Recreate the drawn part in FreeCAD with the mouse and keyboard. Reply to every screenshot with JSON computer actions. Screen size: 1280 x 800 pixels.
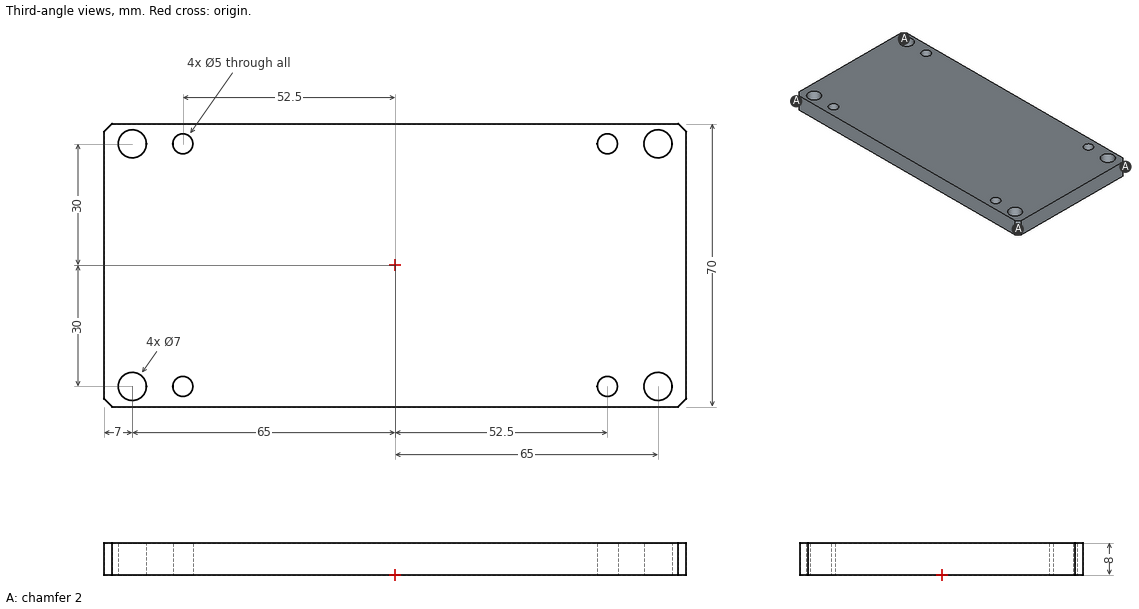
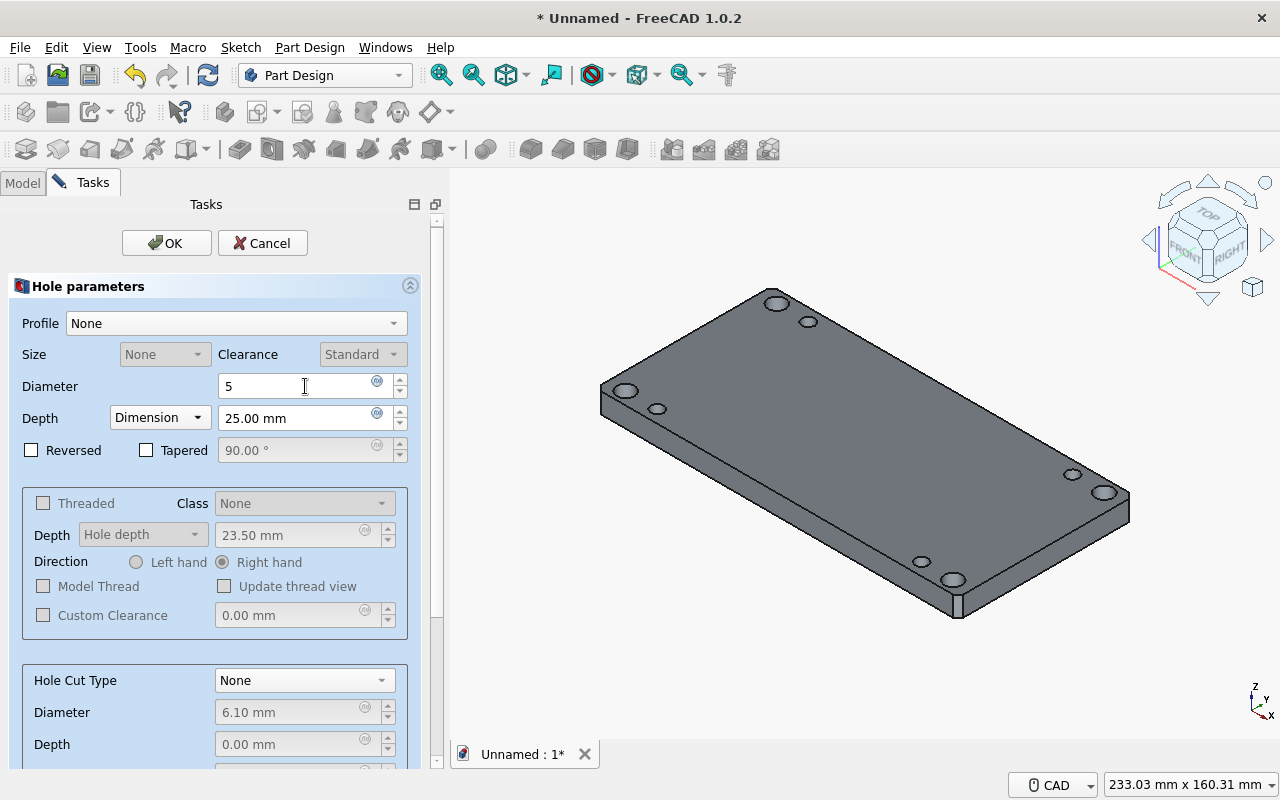
{"action": "left_click", "coordinate": [161, 418]}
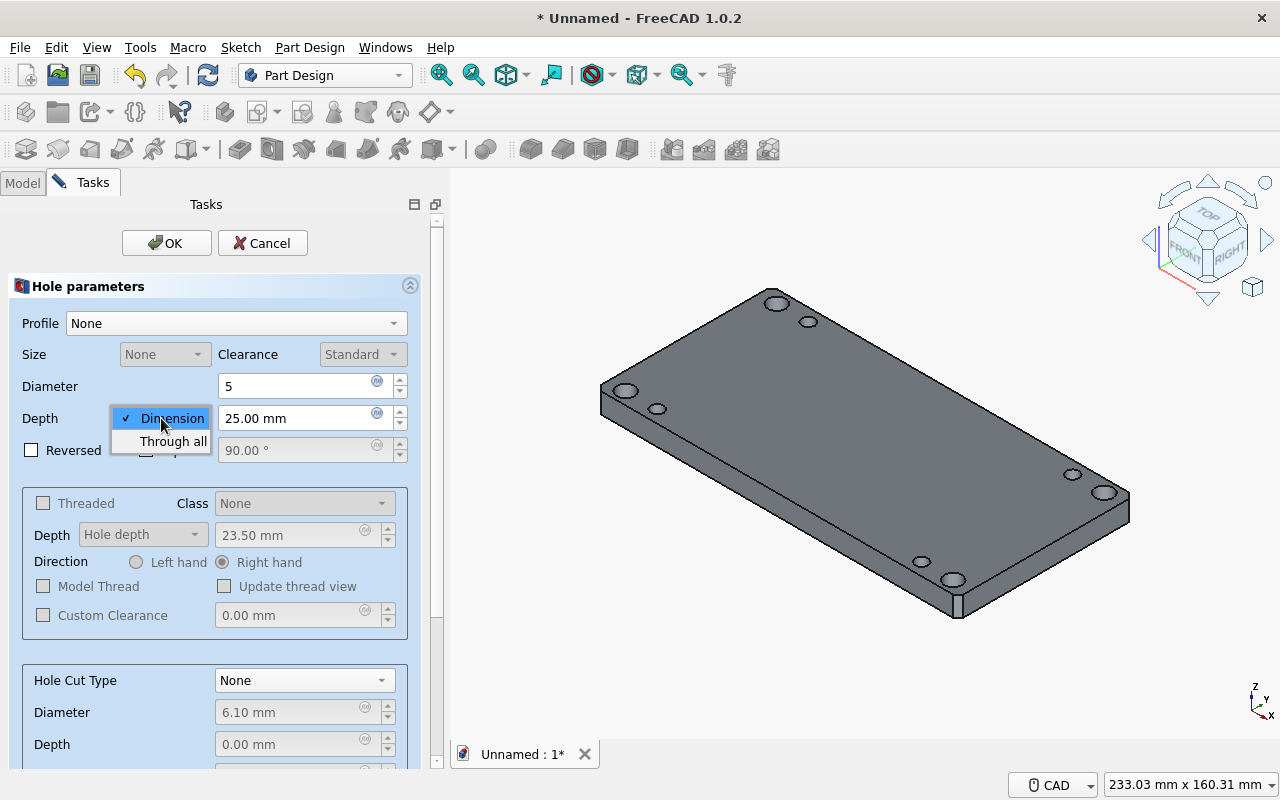
{"action": "left_click", "coordinate": [160, 442]}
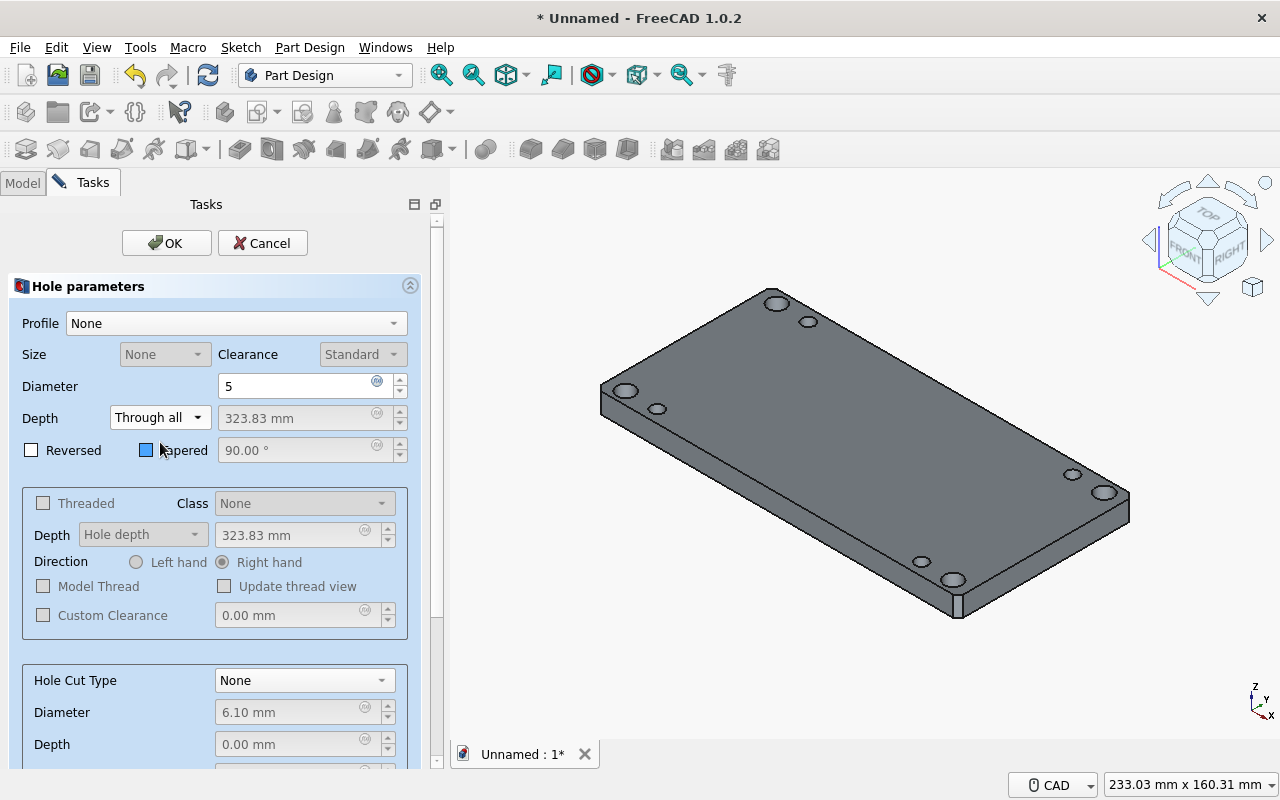
{"action": "left_click", "coordinate": [167, 243]}